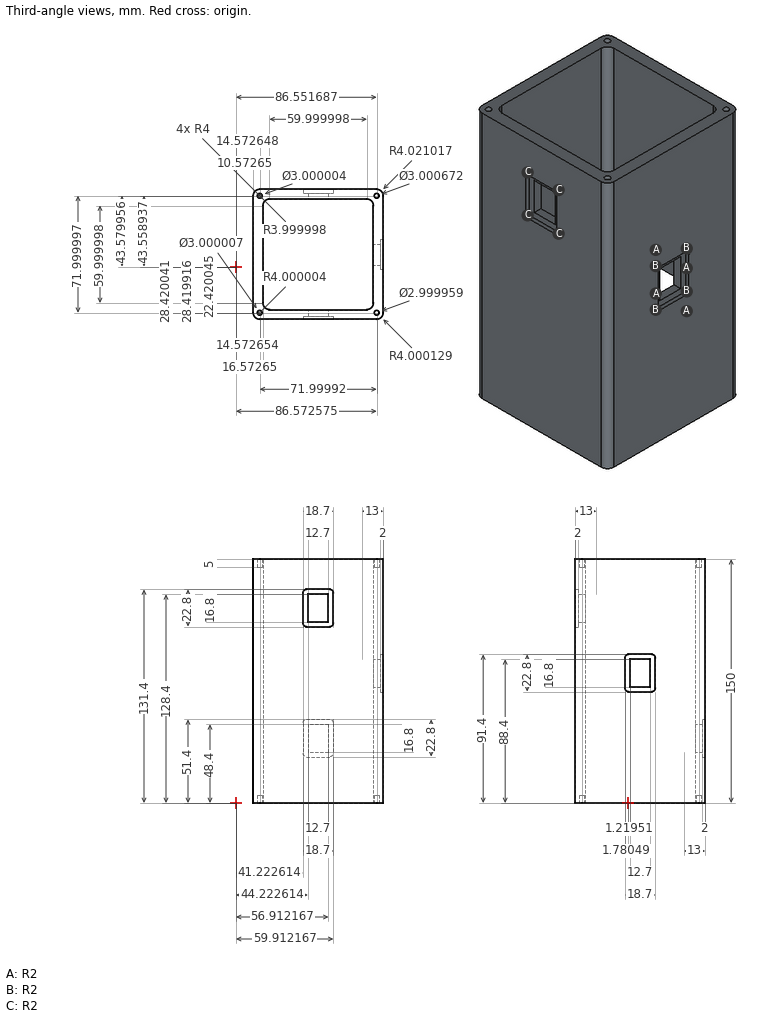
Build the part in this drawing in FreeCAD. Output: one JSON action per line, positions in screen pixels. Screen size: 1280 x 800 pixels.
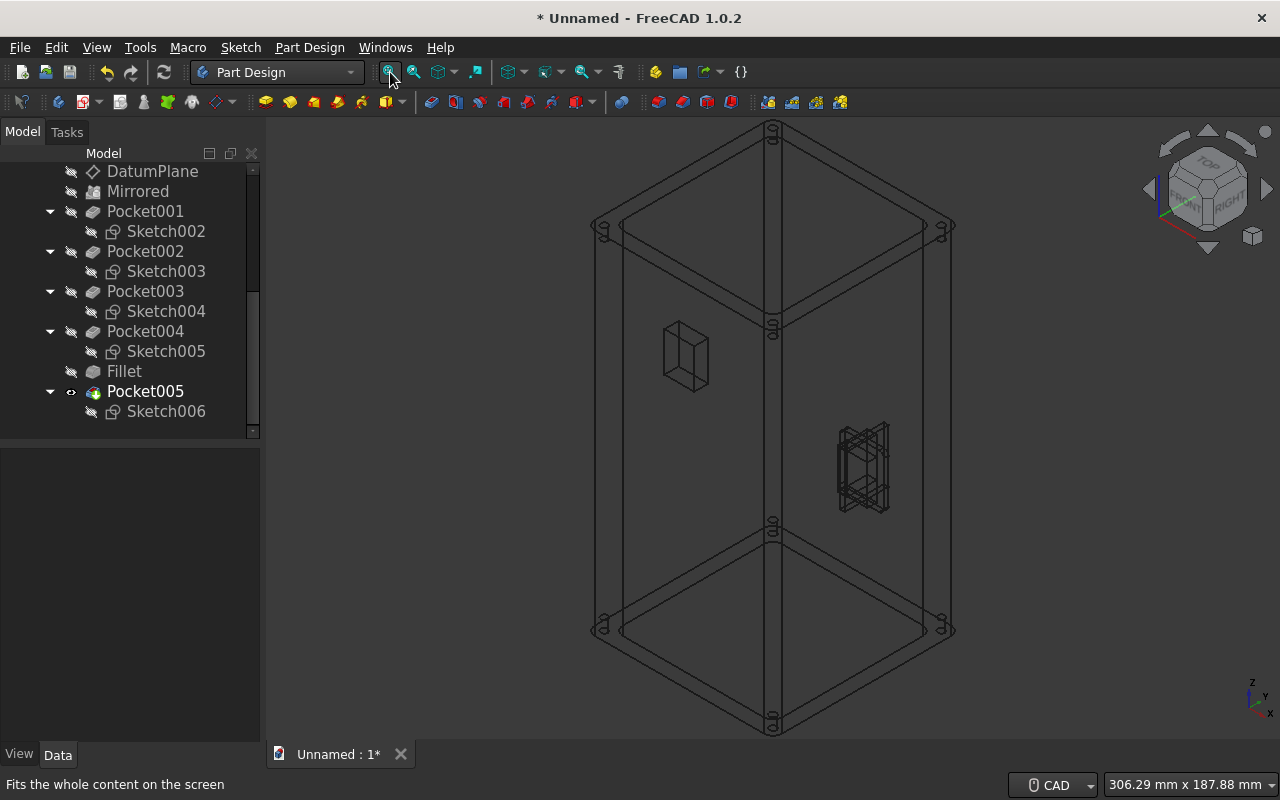
{"action": "key", "text": "v f"}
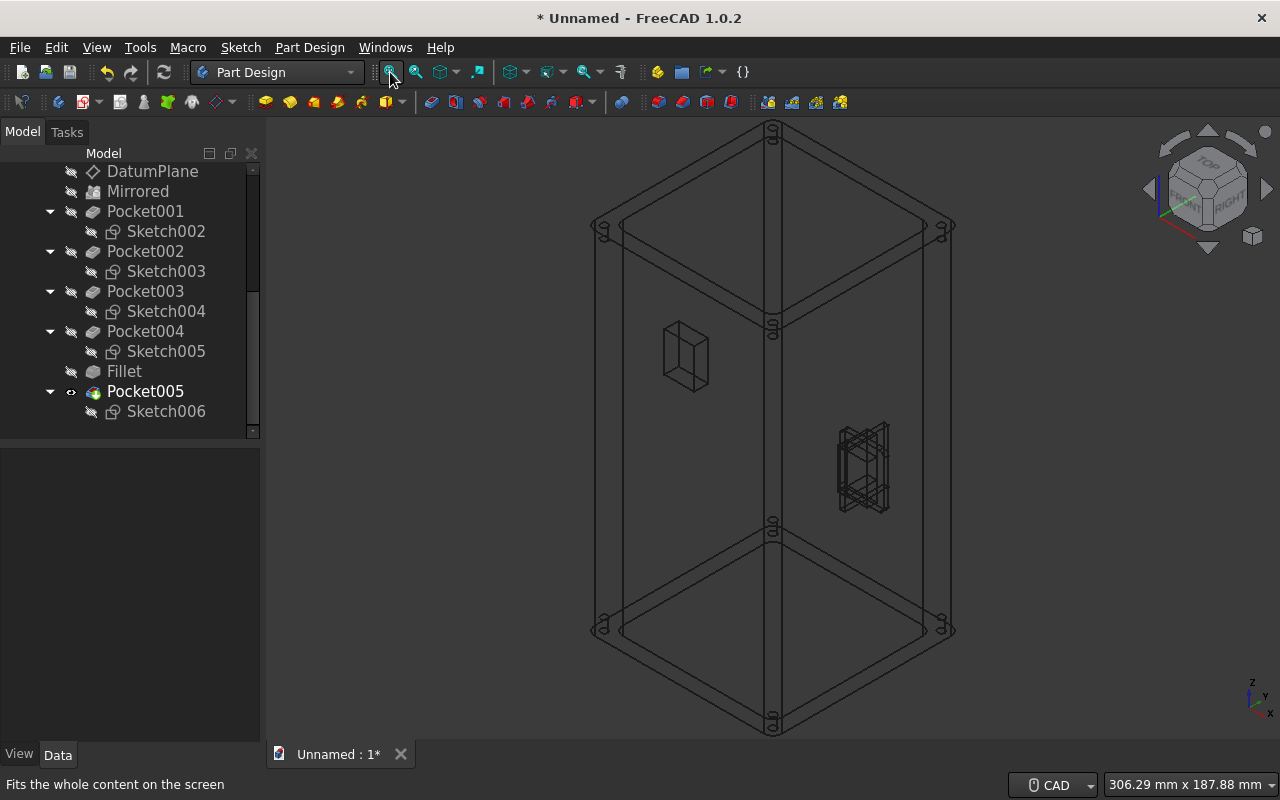
{"action": "scroll", "coordinate": [886, 423], "scroll_direction": "up", "scroll_amount": 9}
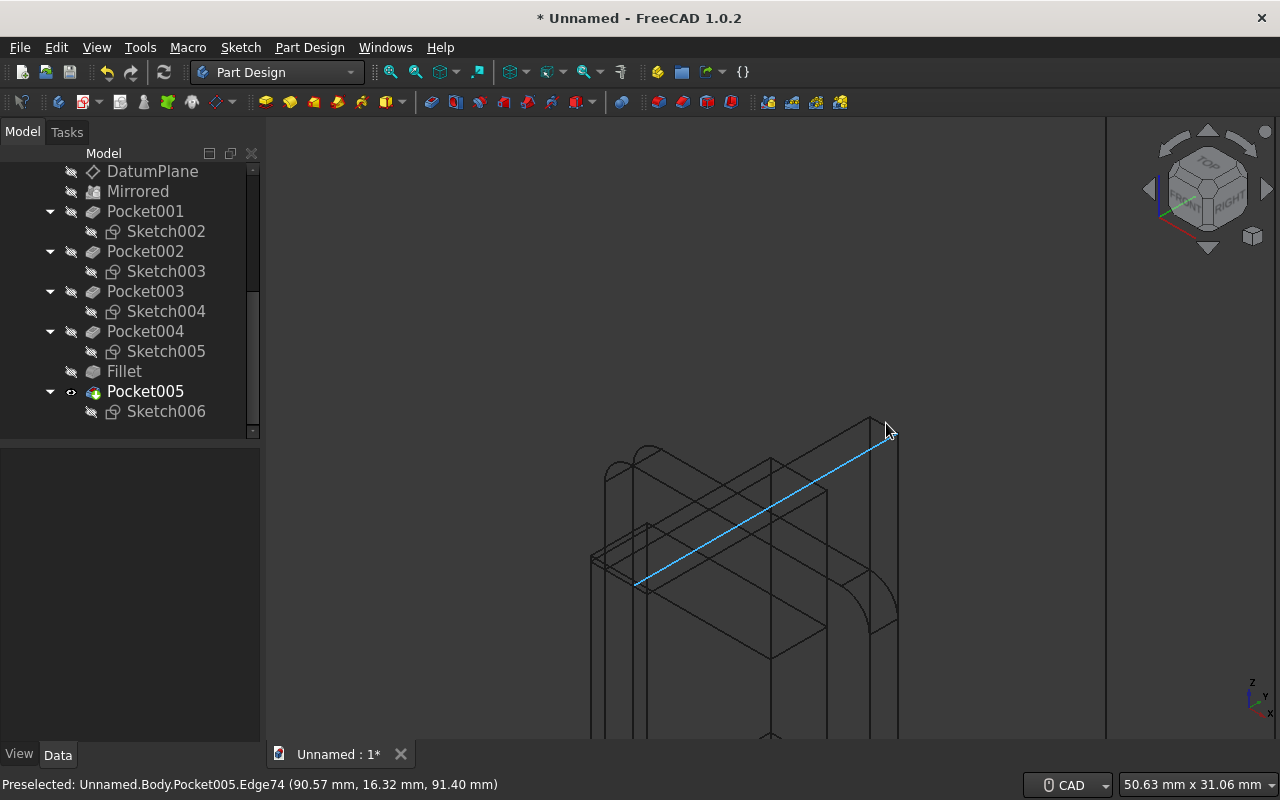
{"action": "left_click", "coordinate": [884, 424]}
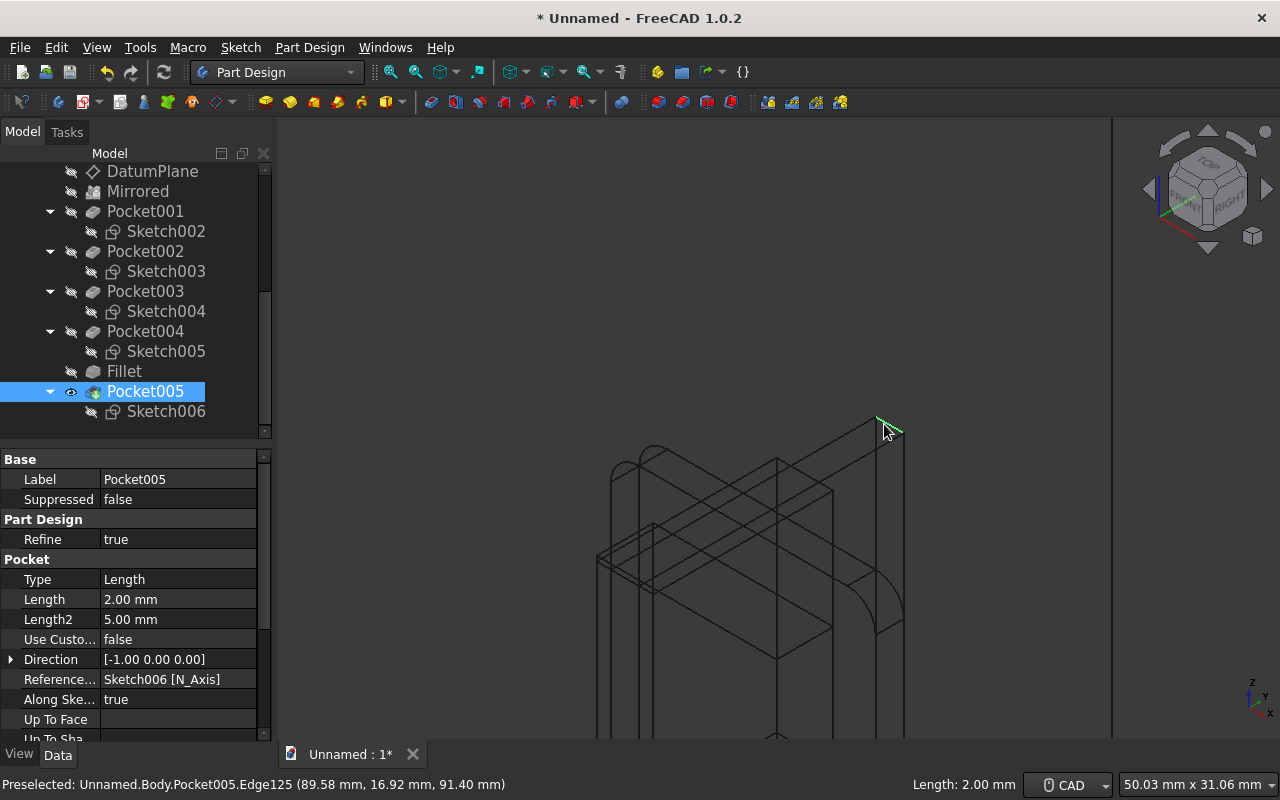
{"action": "left_click", "coordinate": [625, 577], "text": "ctrl"}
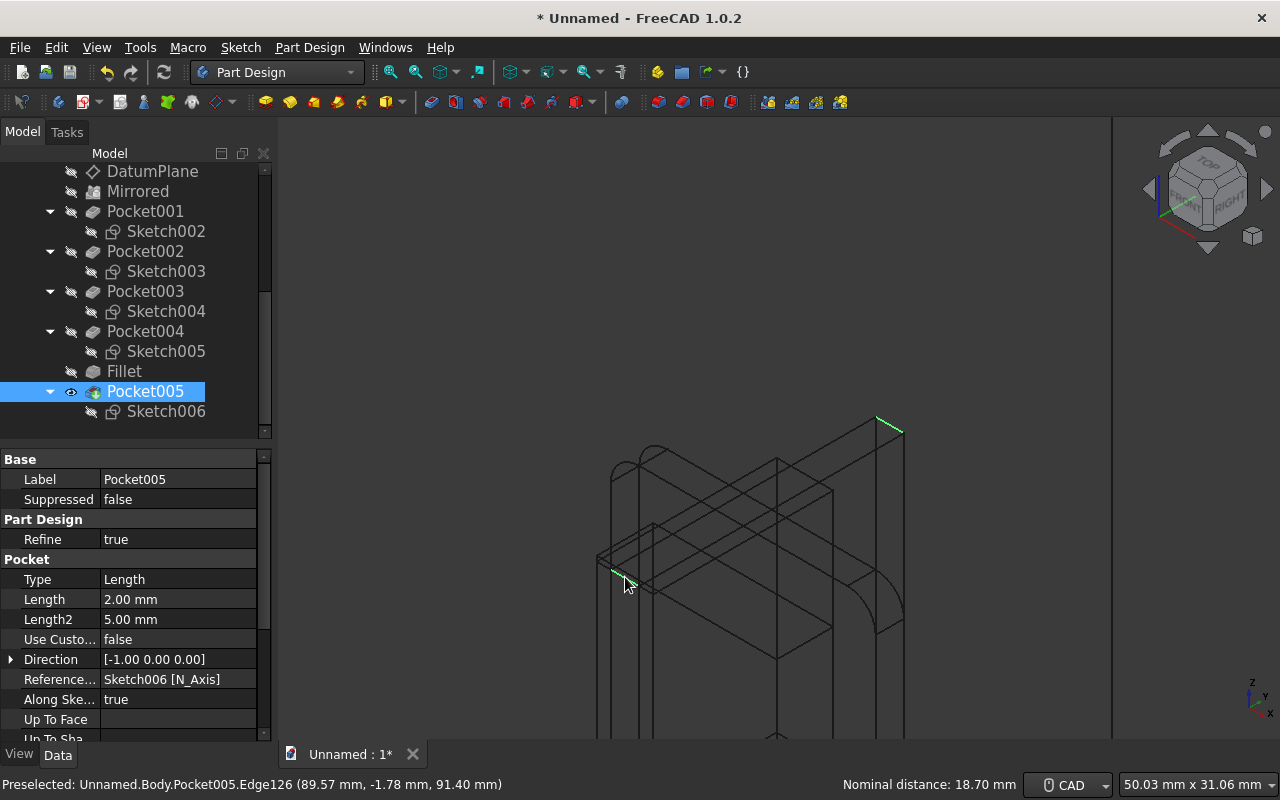
{"action": "left_click", "coordinate": [392, 72]}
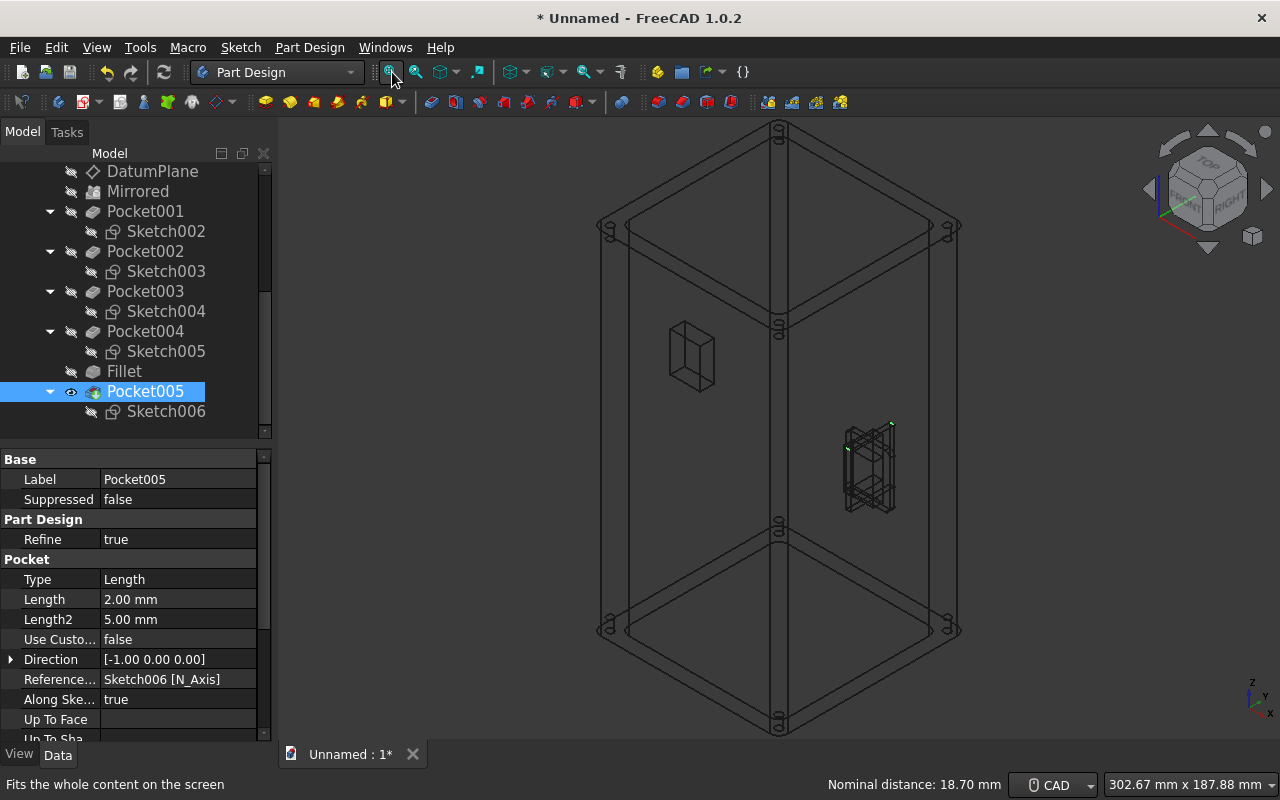
{"action": "key", "text": "2"}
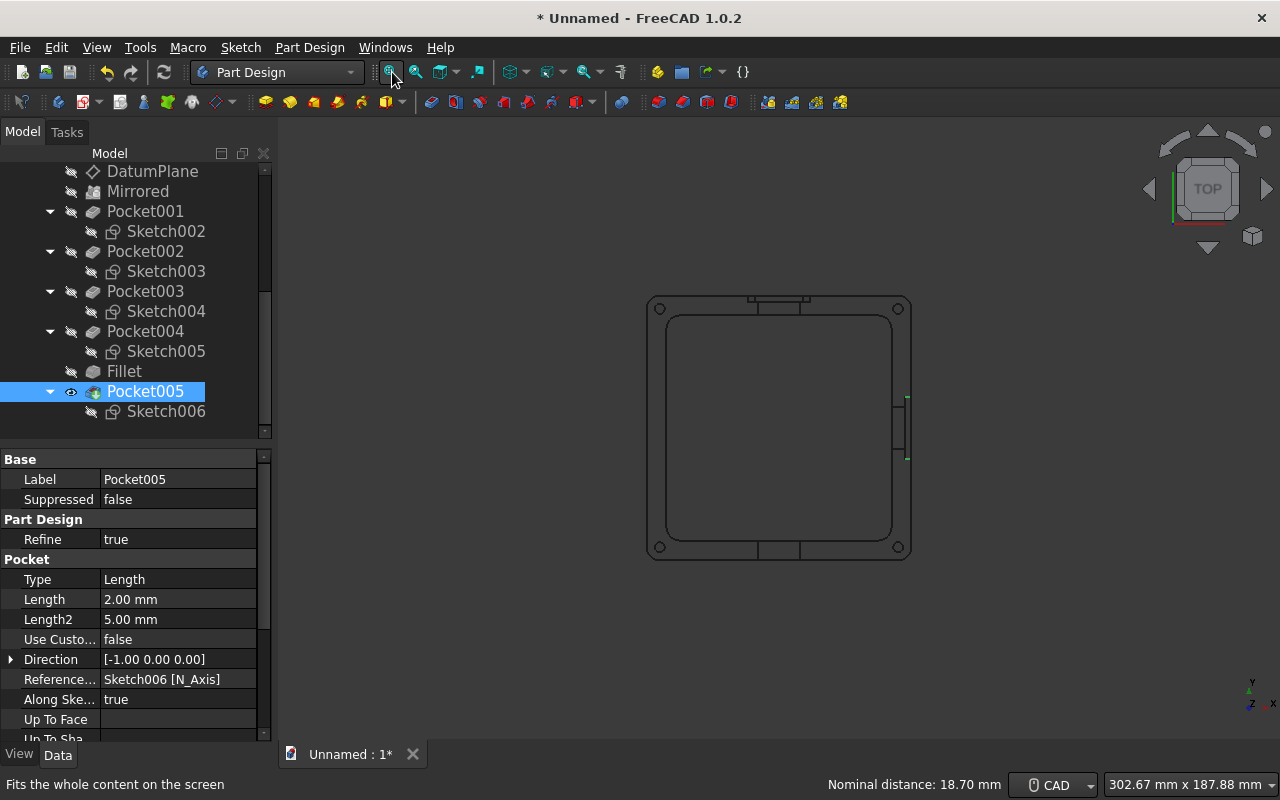
{"action": "left_click", "coordinate": [392, 72]}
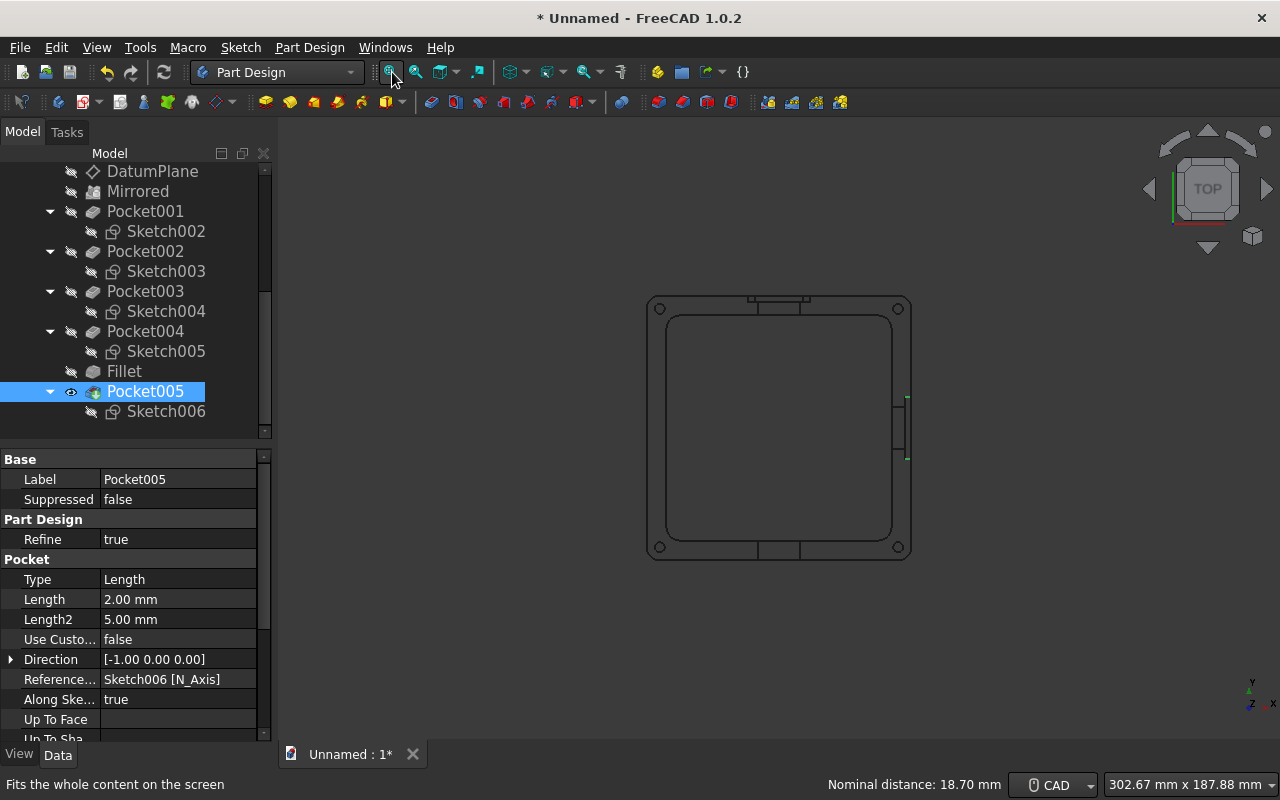
{"action": "scroll", "coordinate": [908, 396], "scroll_direction": "up", "scroll_amount": 9}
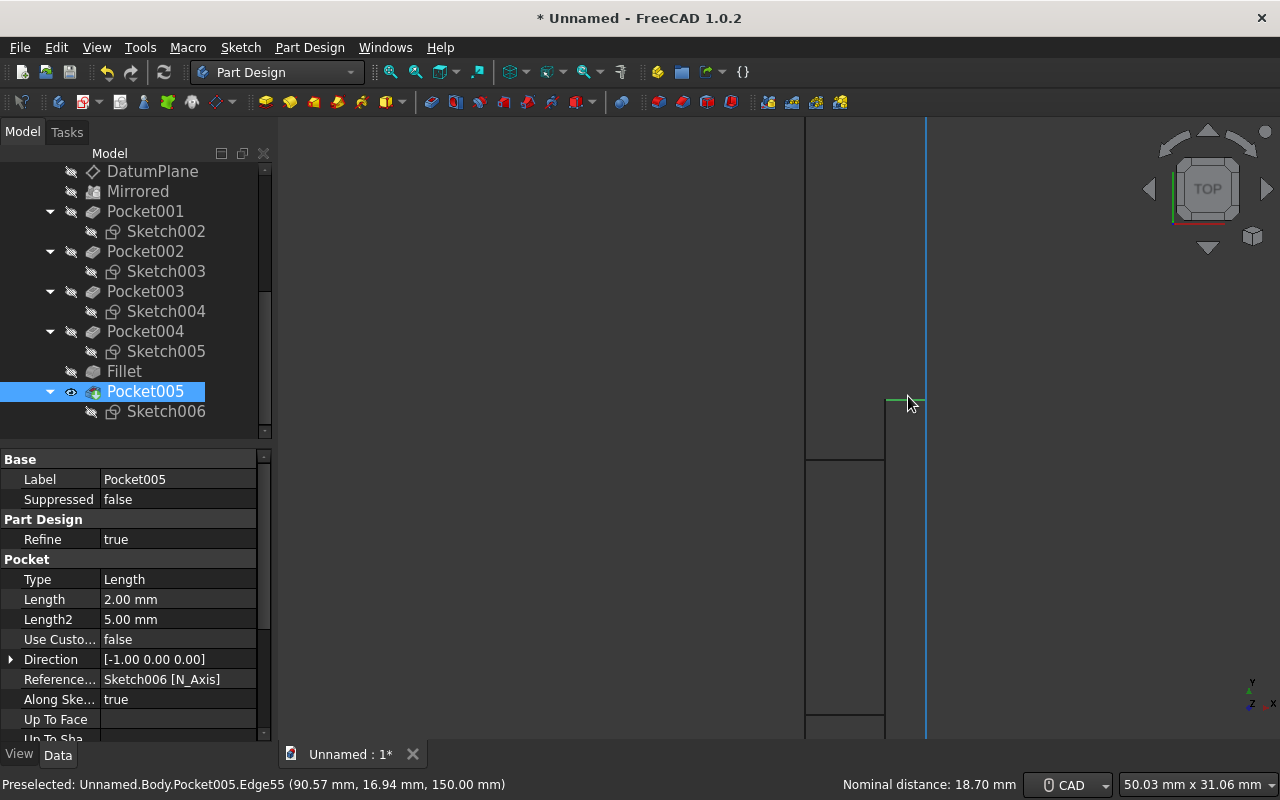
{"action": "left_click", "coordinate": [392, 72]}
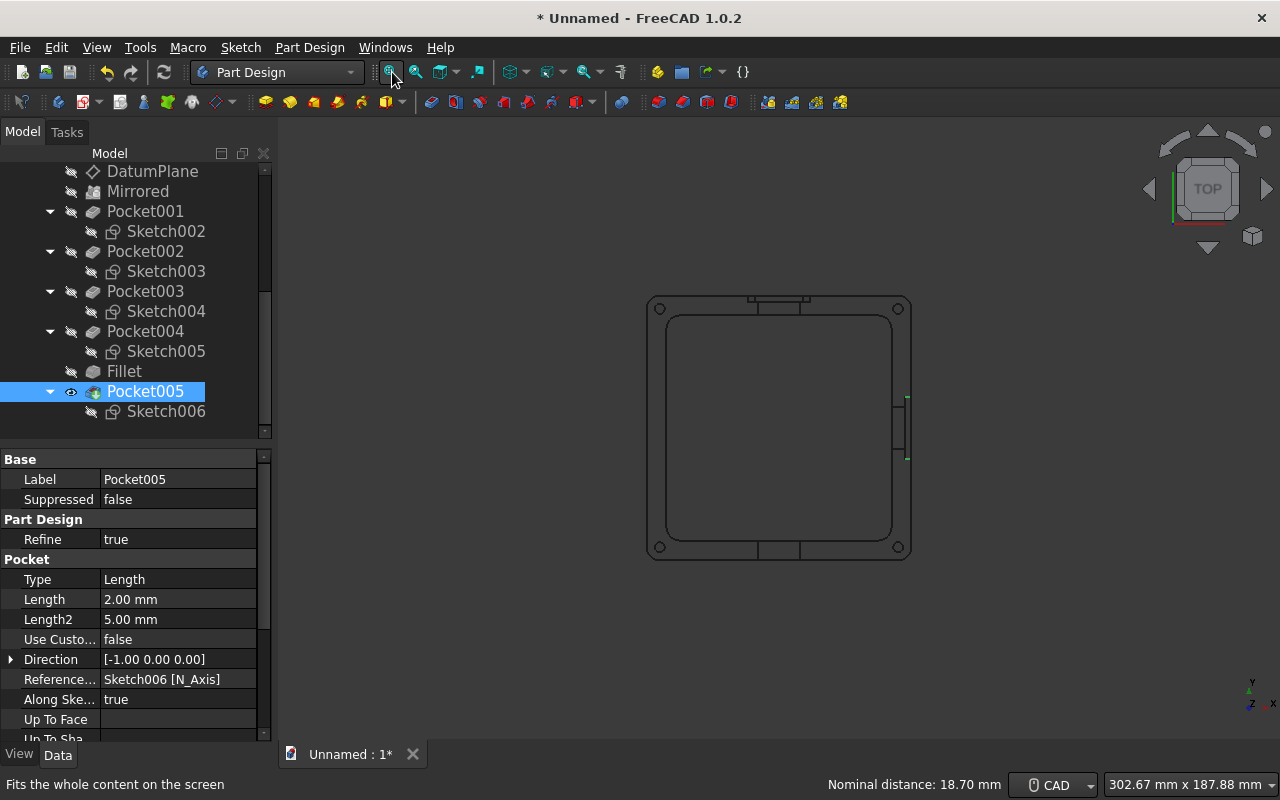
{"action": "key", "text": "1"}